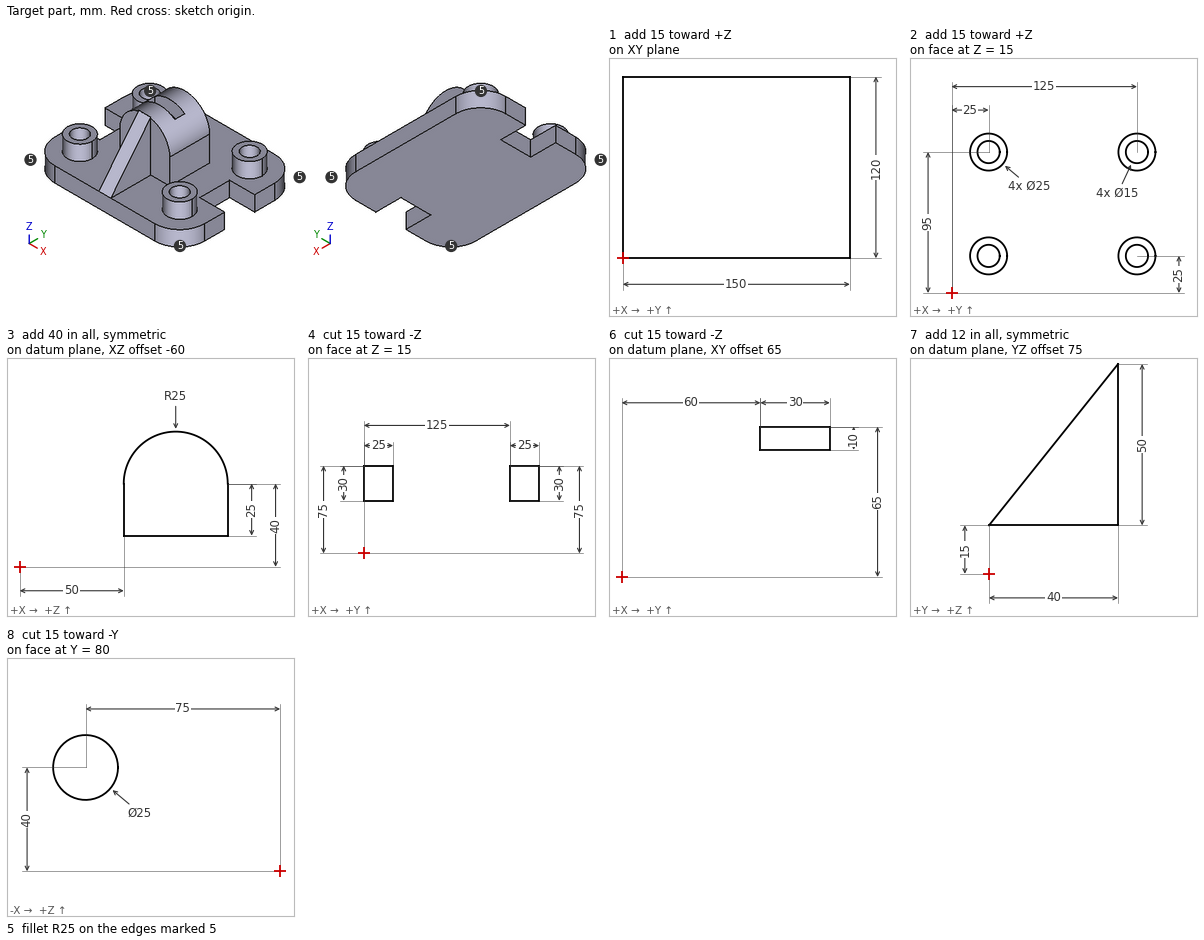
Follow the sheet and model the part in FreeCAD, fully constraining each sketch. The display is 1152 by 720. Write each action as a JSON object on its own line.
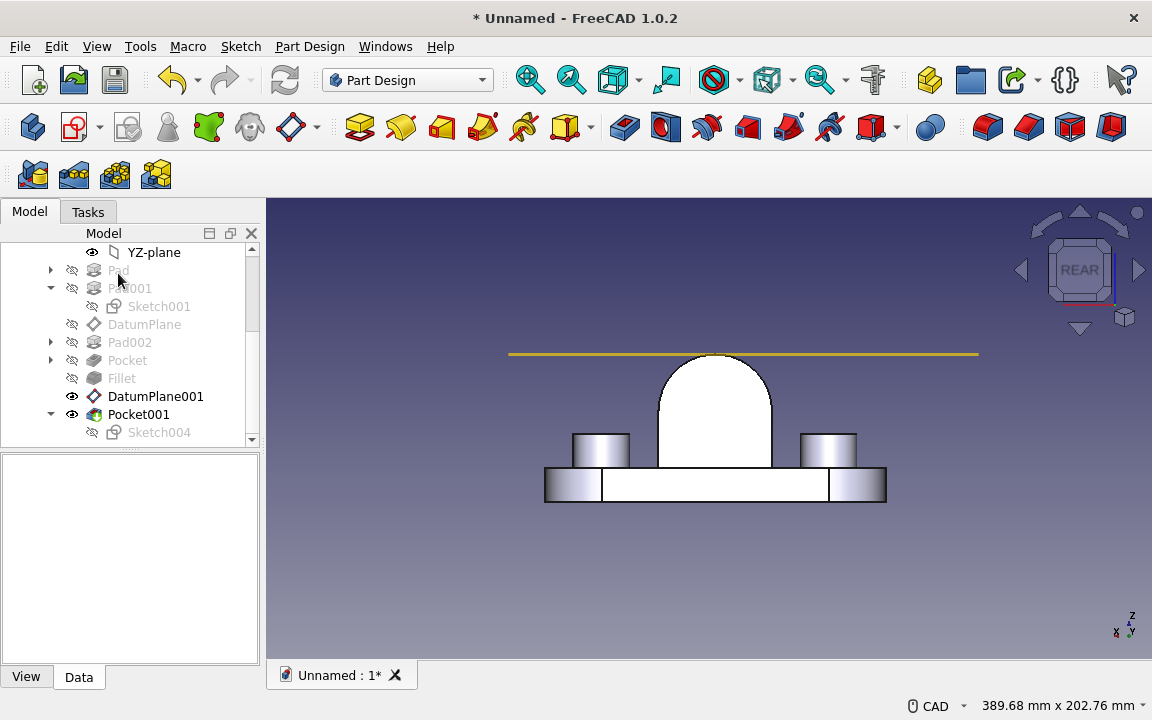
{"action": "left_click", "coordinate": [117, 396]}
{"action": "key", "text": "space"}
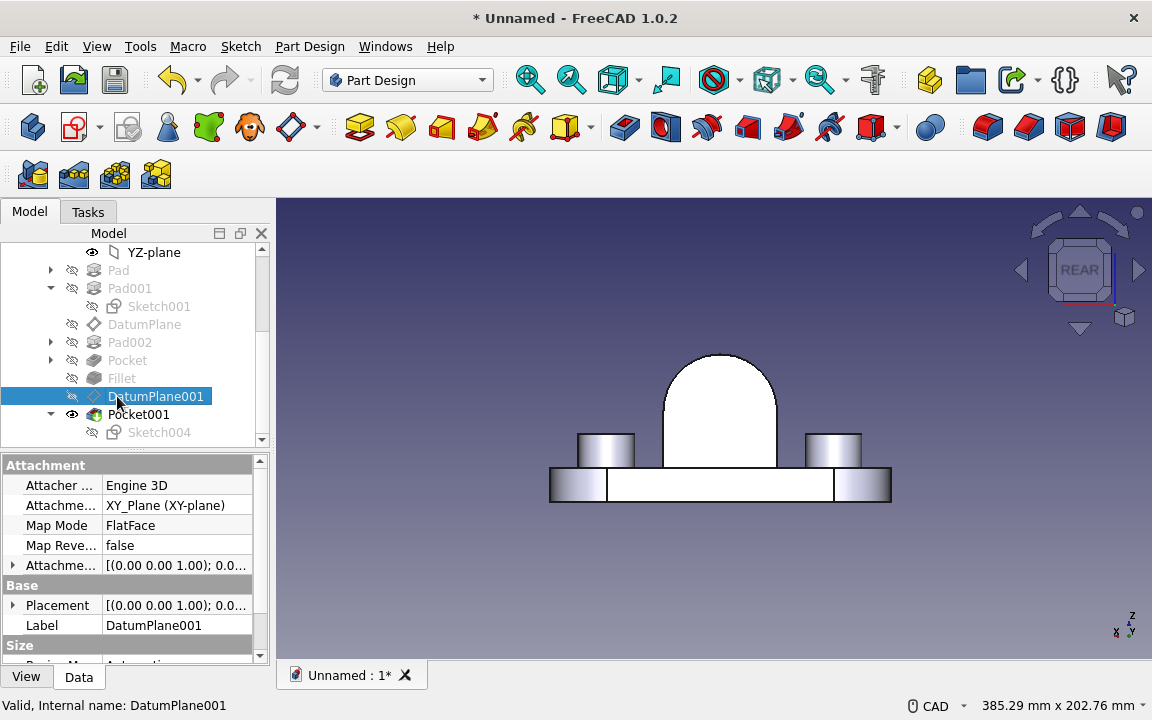
{"action": "left_click", "coordinate": [531, 80]}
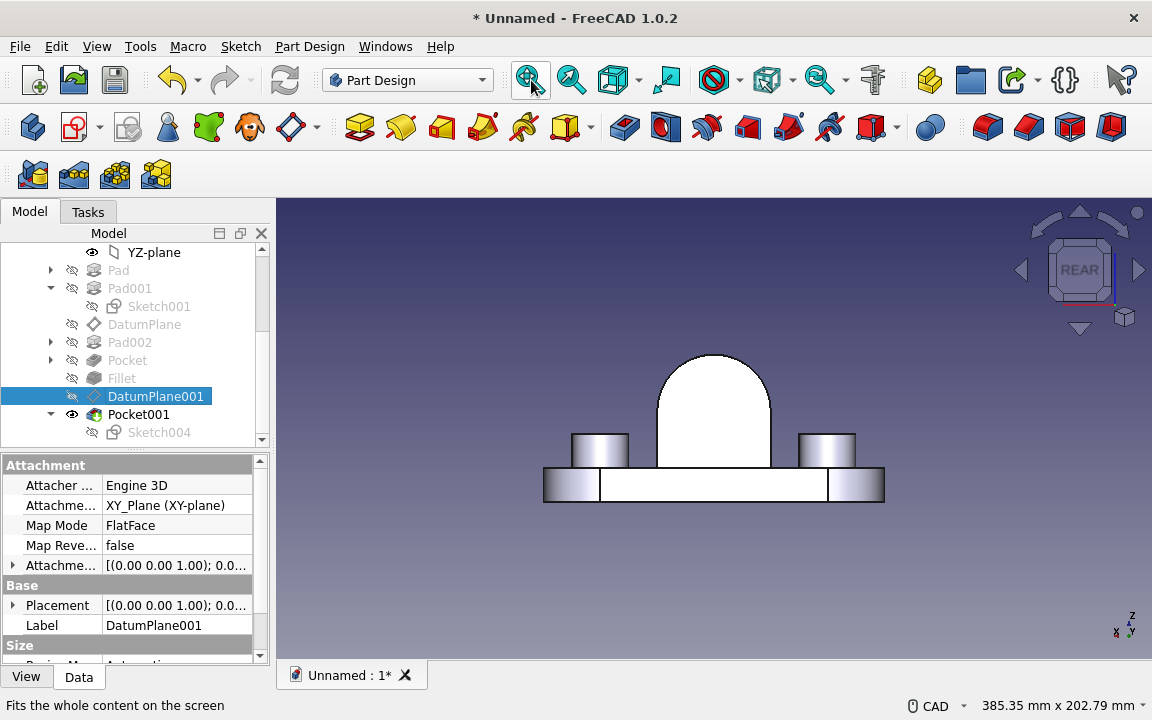
{"action": "scroll", "coordinate": [161, 338], "scroll_direction": "down", "scroll_amount": 3}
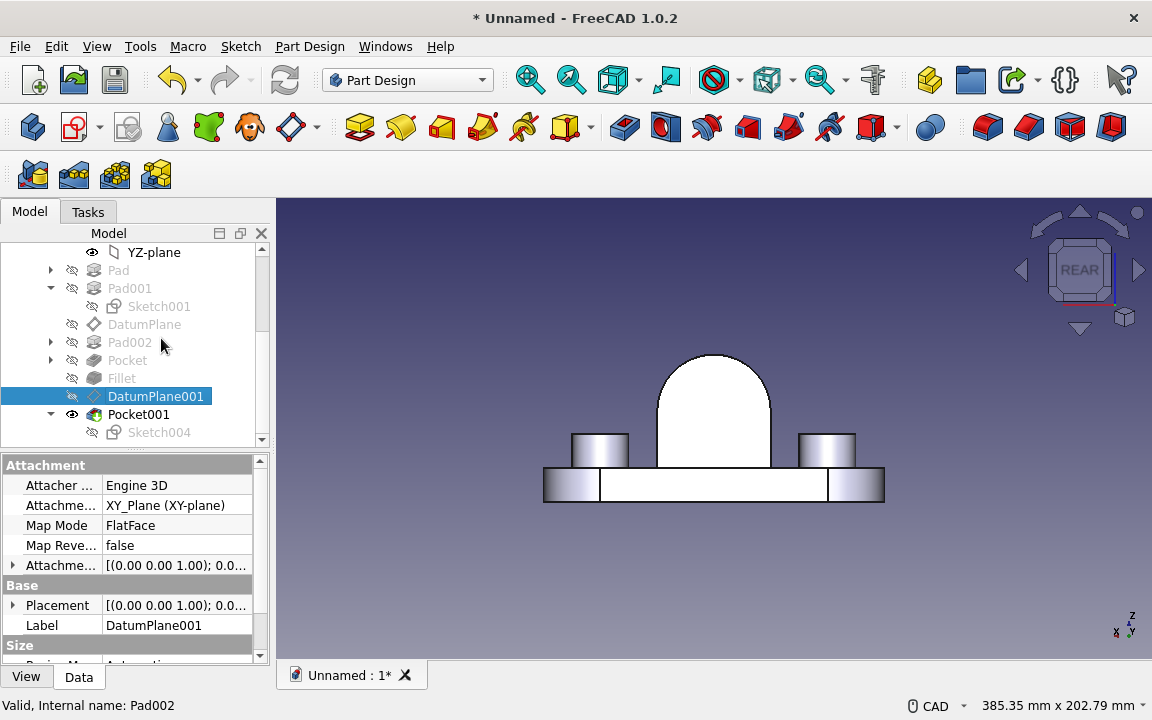
{"action": "scroll", "coordinate": [161, 338], "scroll_direction": "up", "scroll_amount": 15}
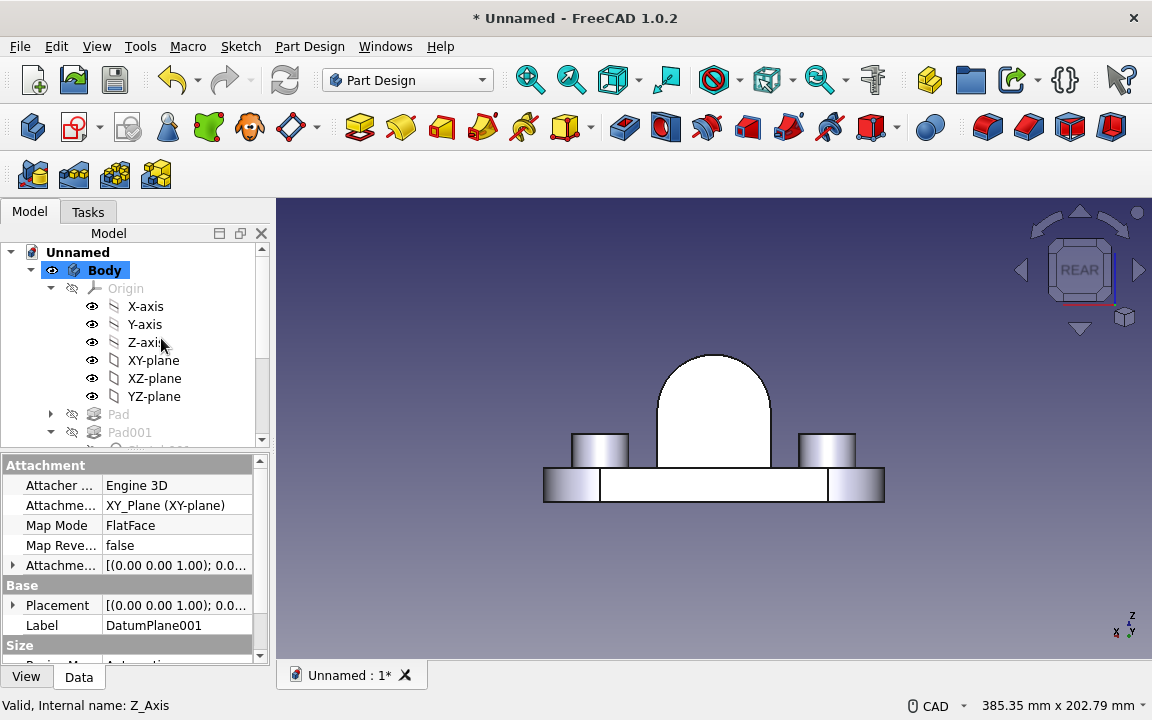
{"action": "left_click", "coordinate": [137, 396]}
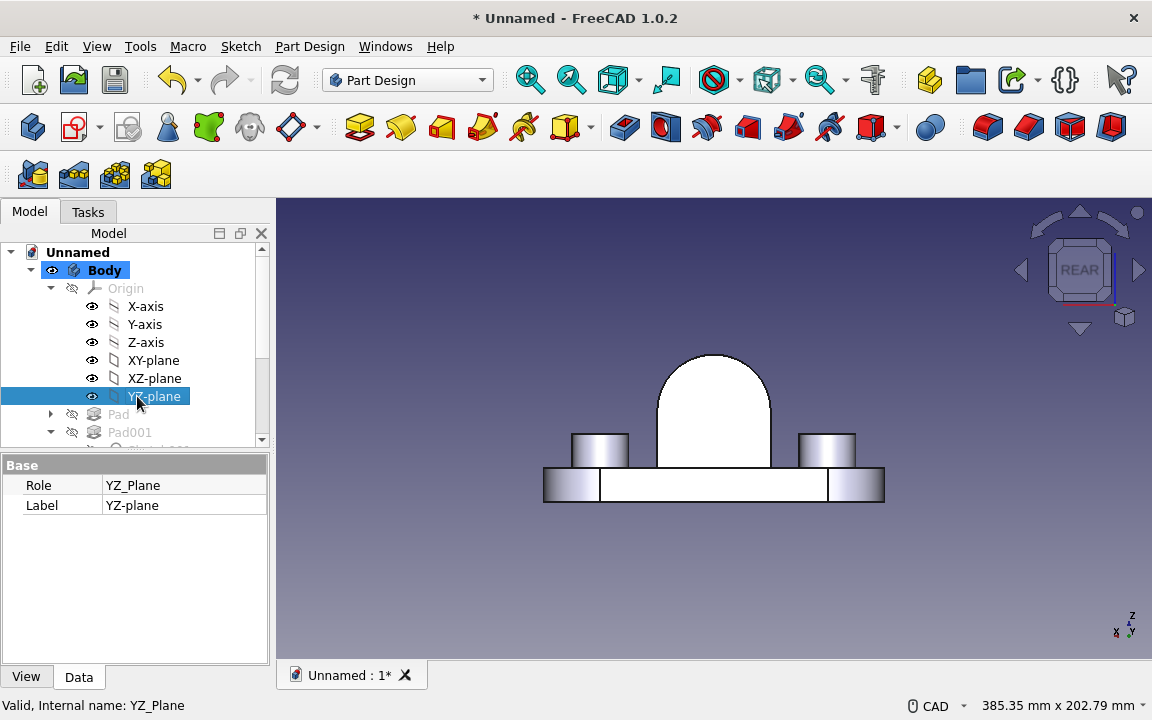
{"action": "left_click", "coordinate": [290, 128]}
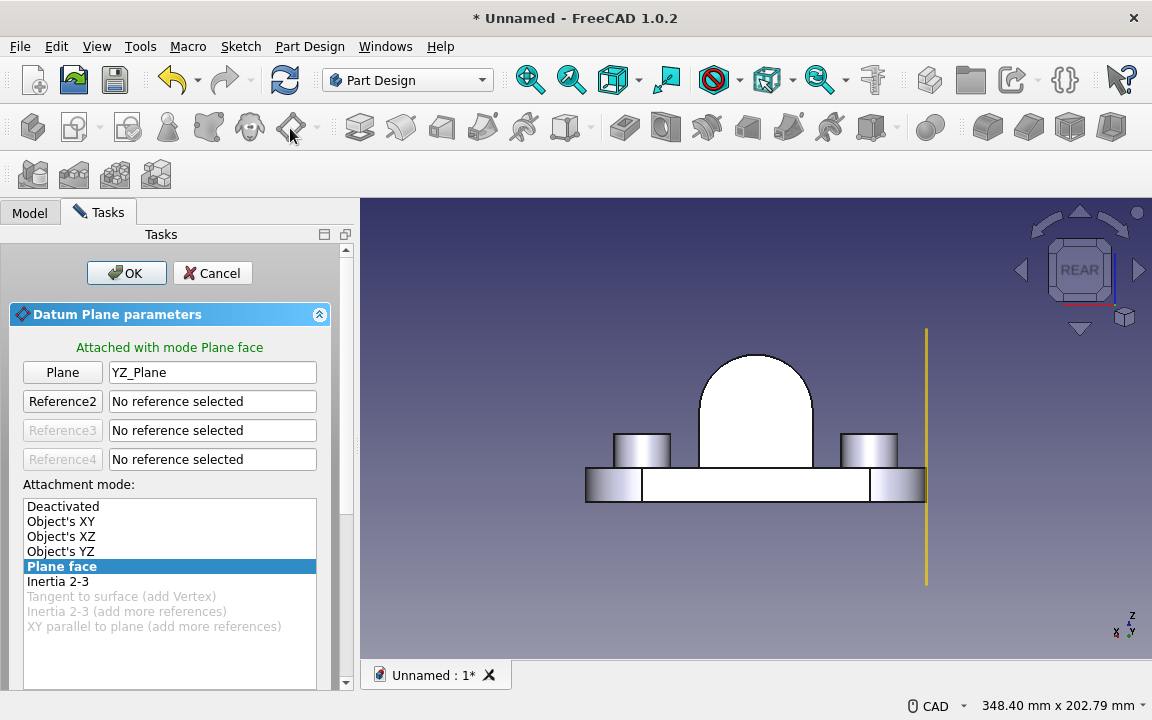
{"action": "scroll", "coordinate": [346, 467], "scroll_direction": "down", "scroll_amount": 4}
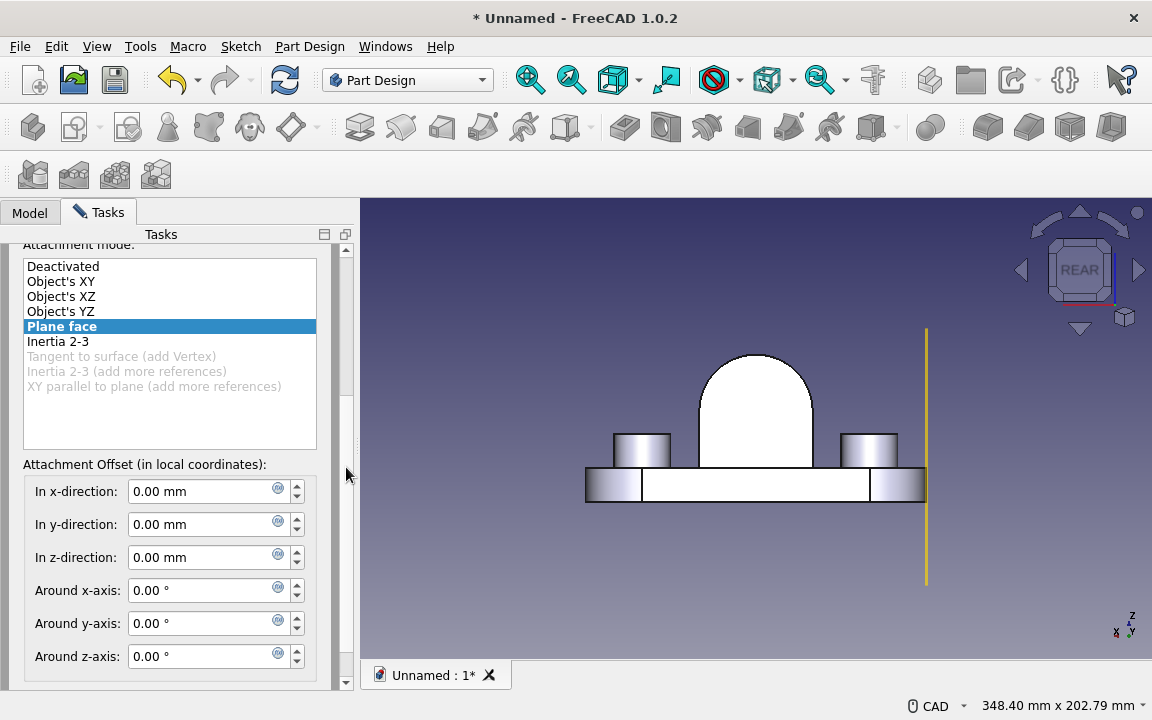
{"action": "triple_click", "coordinate": [210, 558]}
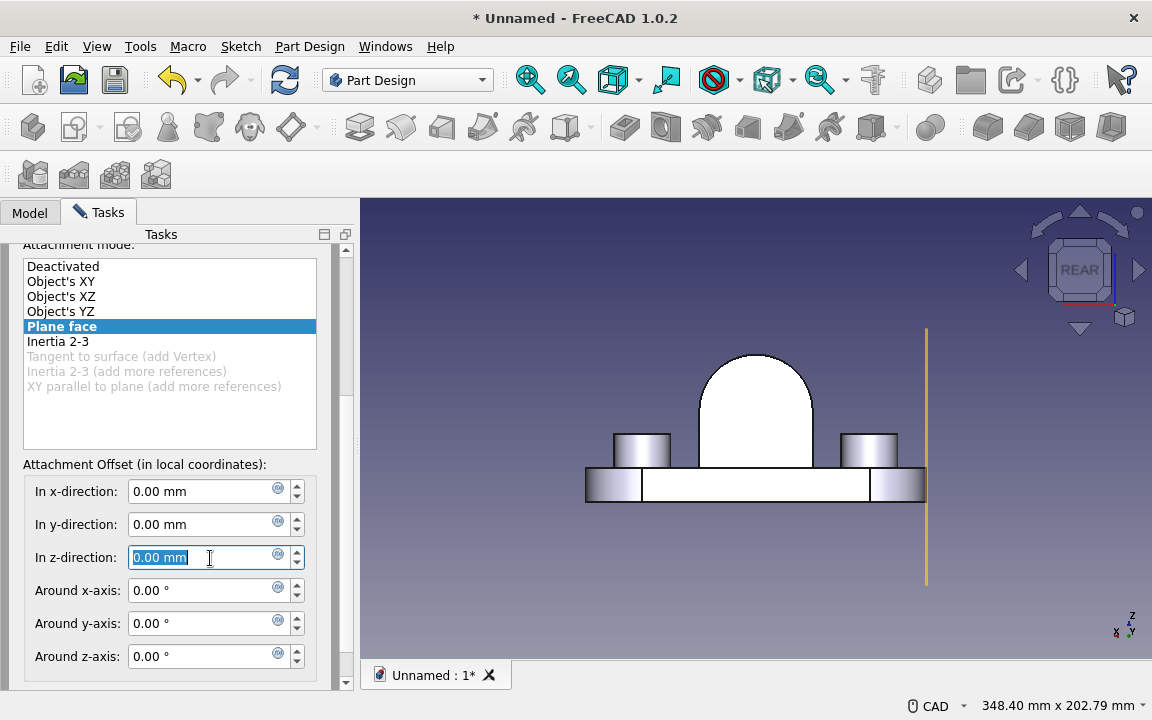
{"action": "type", "text": "75"}
{"action": "key", "text": "Tab"}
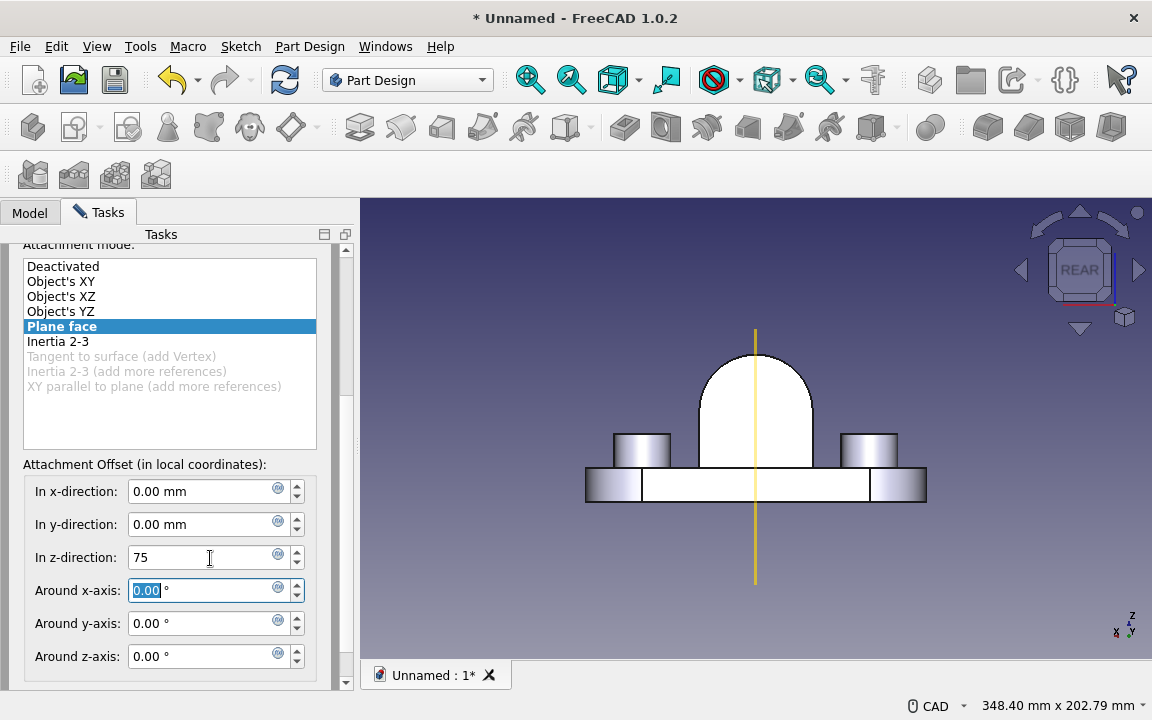
{"action": "scroll", "coordinate": [346, 467], "scroll_direction": "up", "scroll_amount": 5}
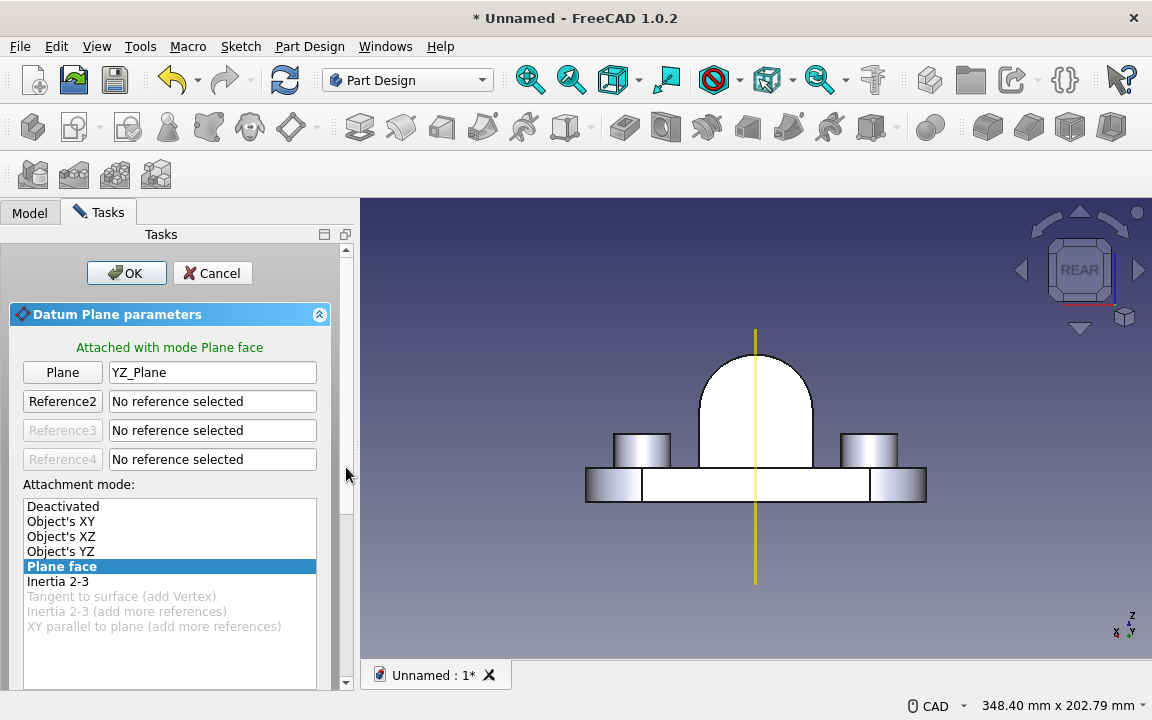
{"action": "left_click", "coordinate": [127, 273]}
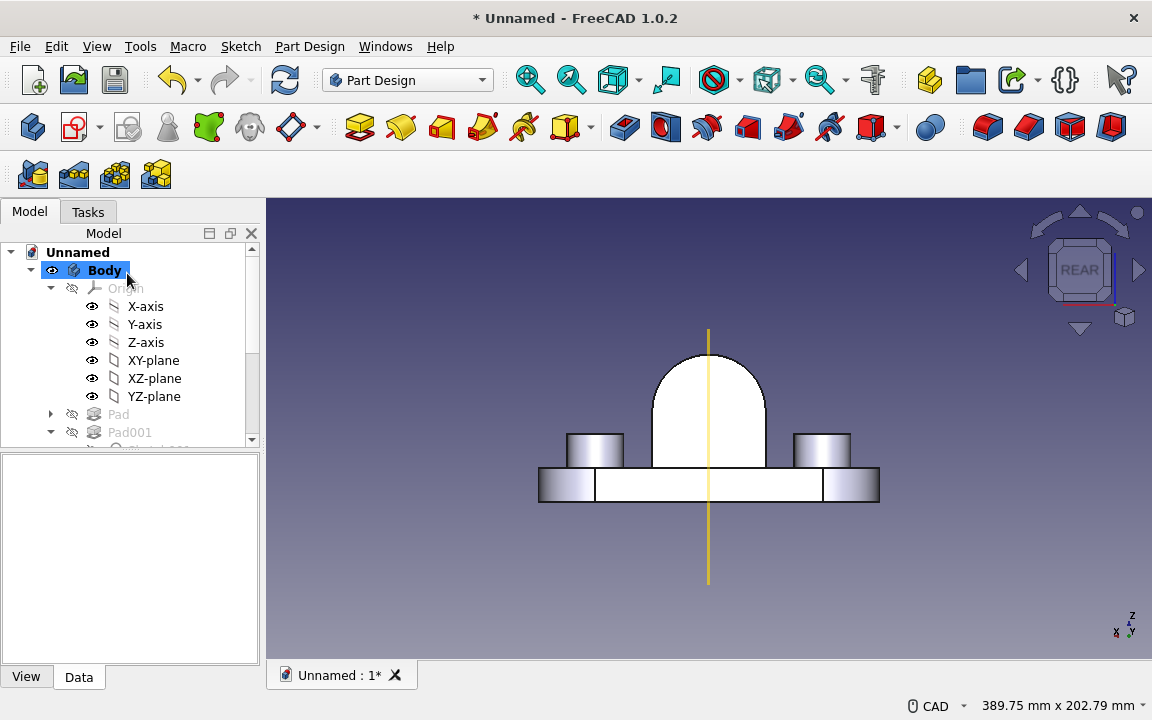
{"action": "scroll", "coordinate": [101, 338], "scroll_direction": "down", "scroll_amount": 3}